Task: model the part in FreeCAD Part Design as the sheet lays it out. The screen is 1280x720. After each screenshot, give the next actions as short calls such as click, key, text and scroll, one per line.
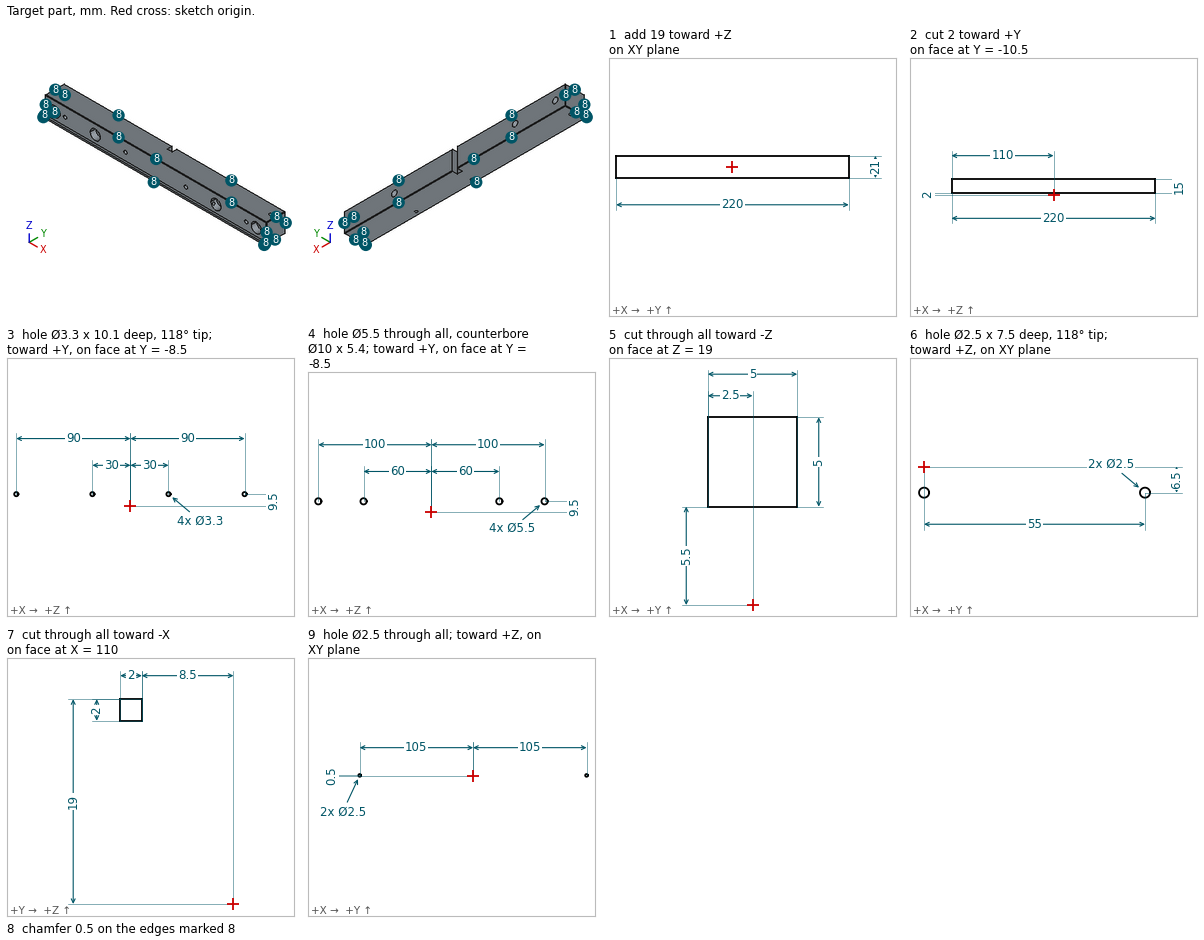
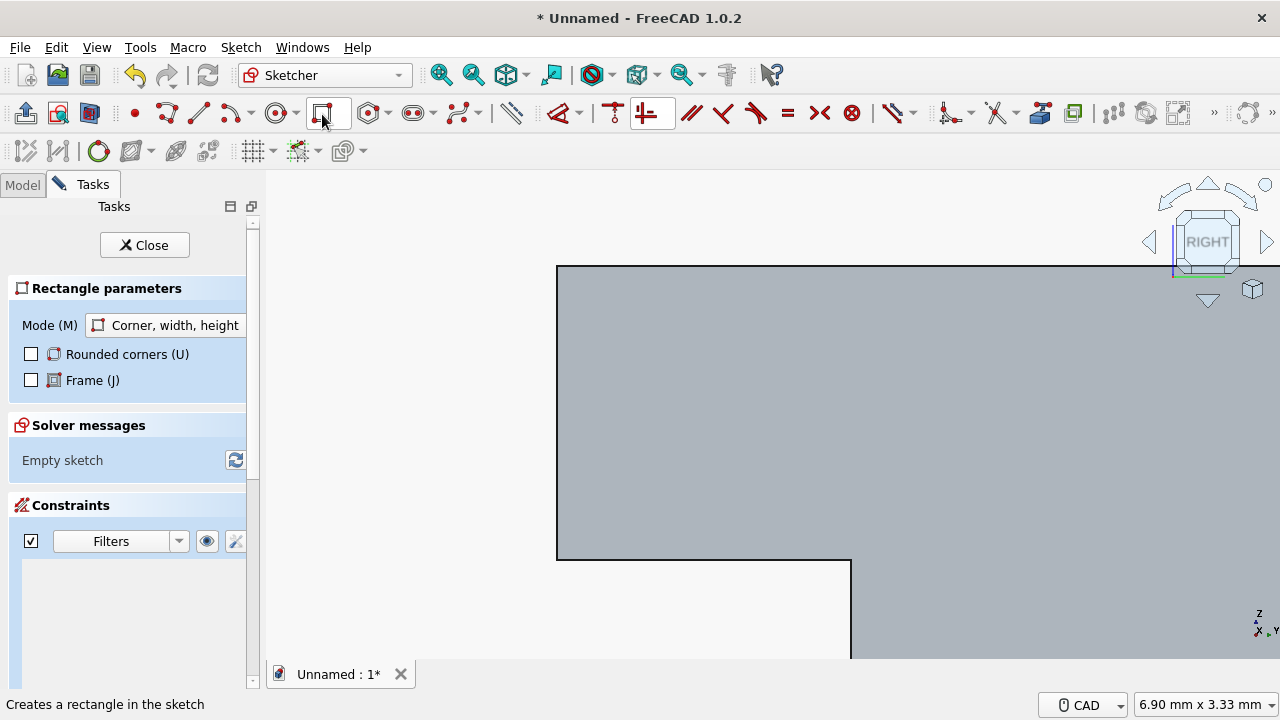
click(557, 266)
move(851, 560)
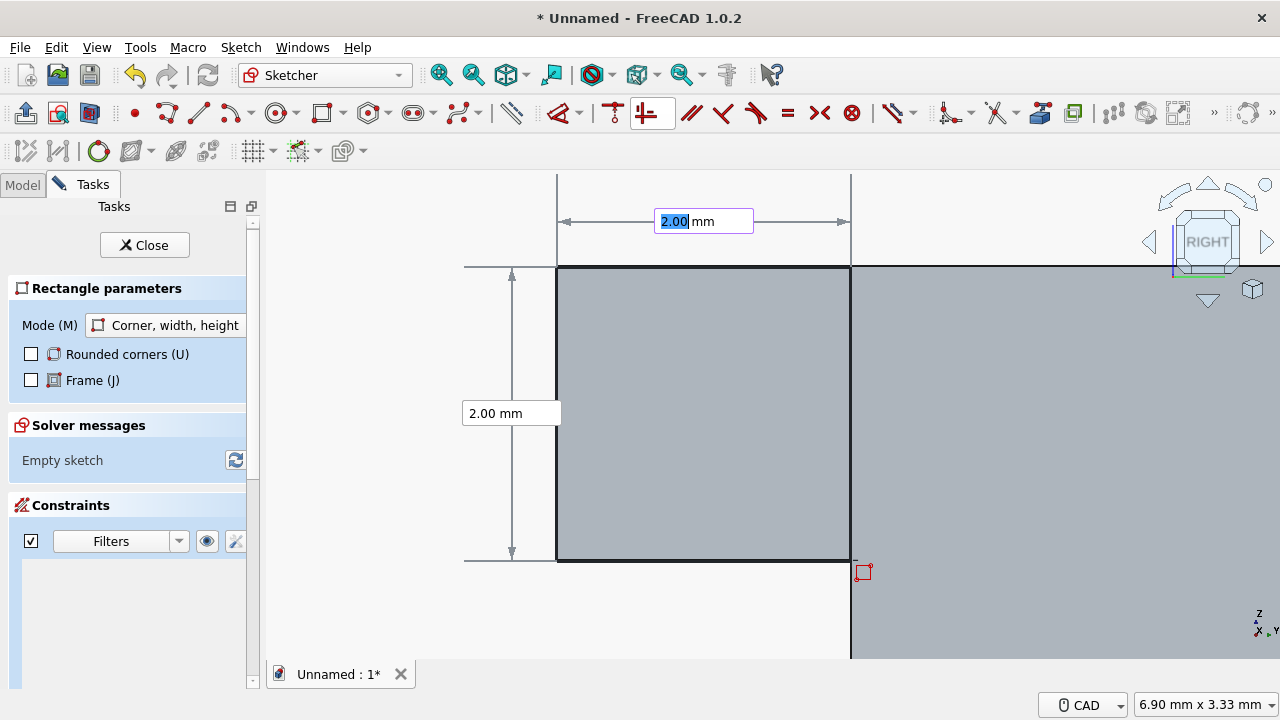
text(2)
key(Tab)
text(2)
key(Return)
key(Escape)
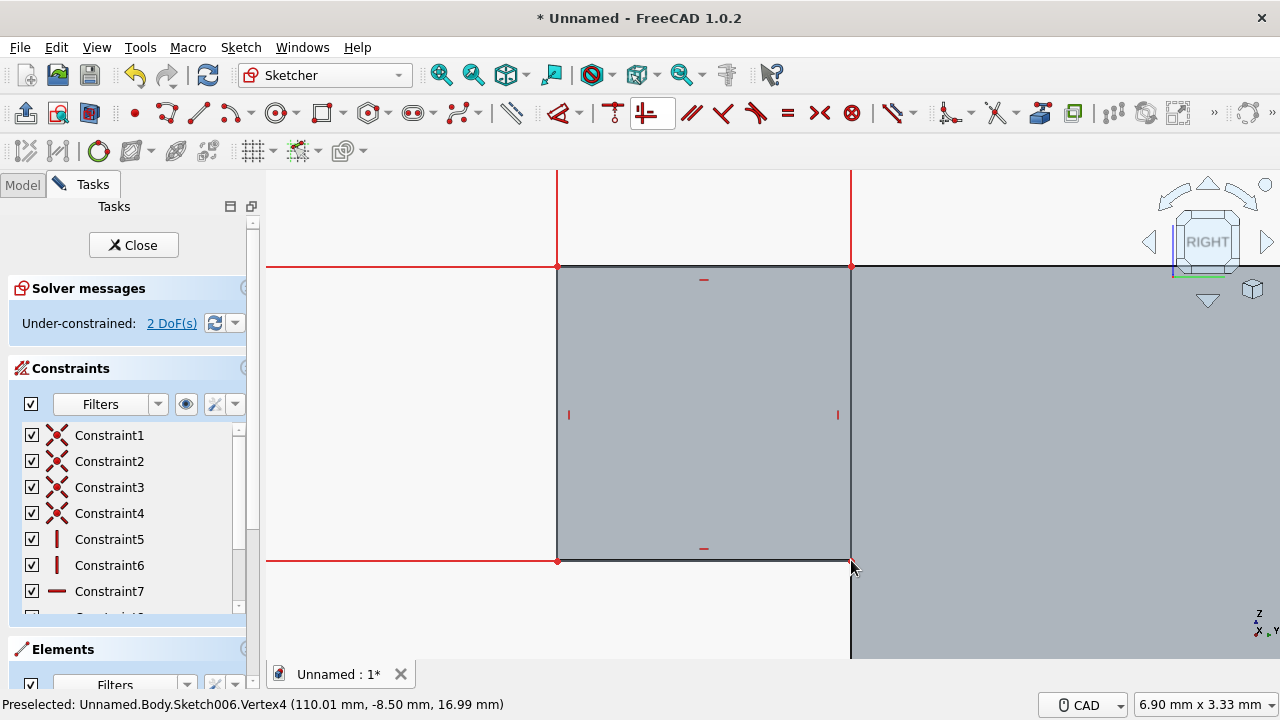
click(558, 114)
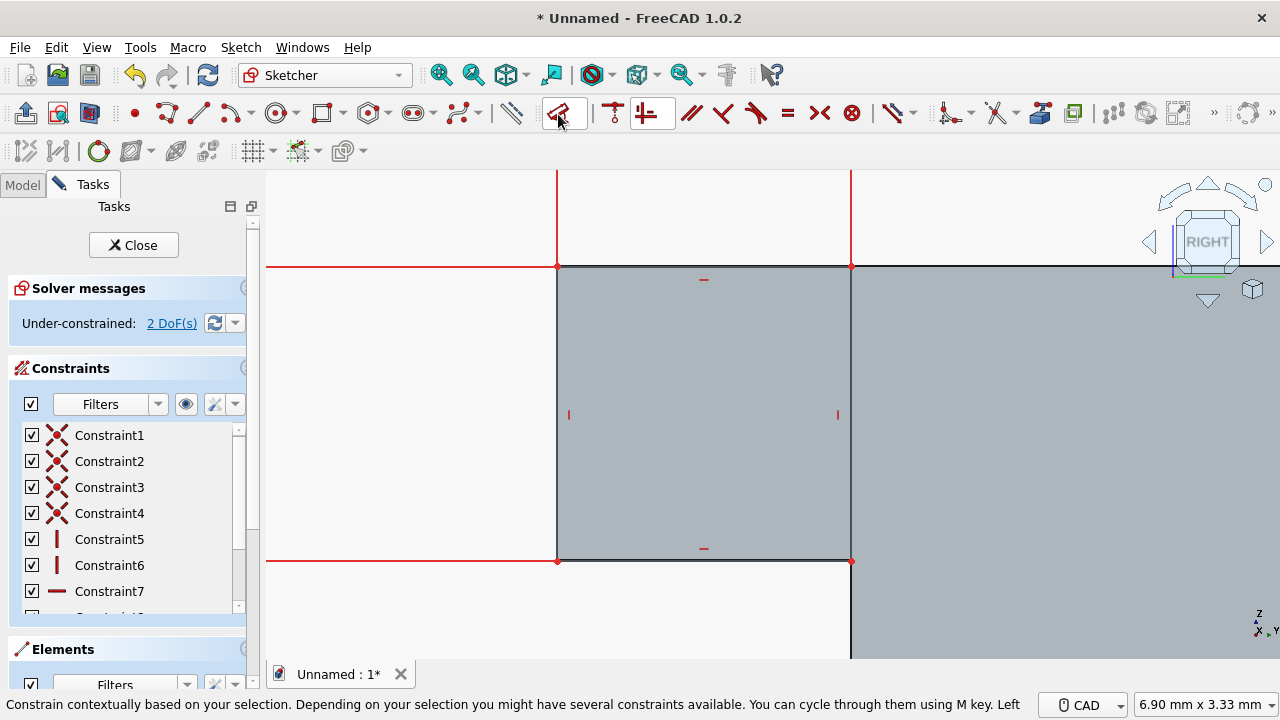
click(557, 267)
click(523, 449)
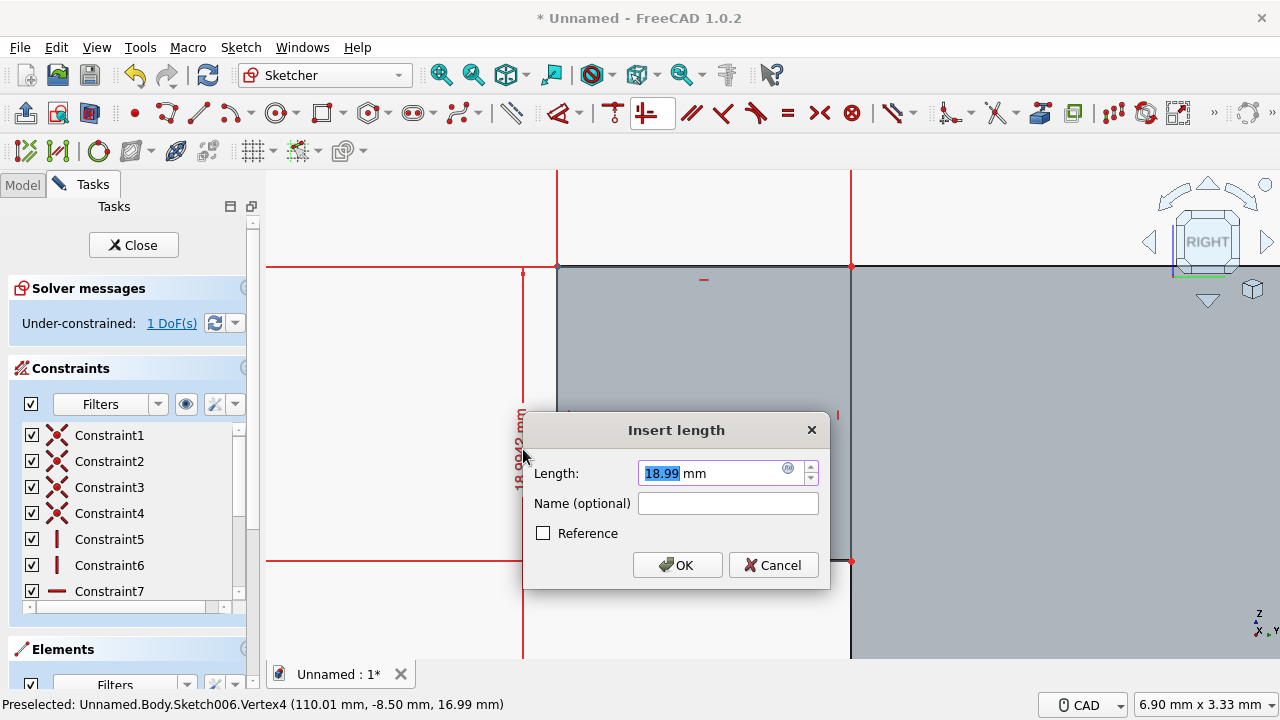
text(19)
key(Return)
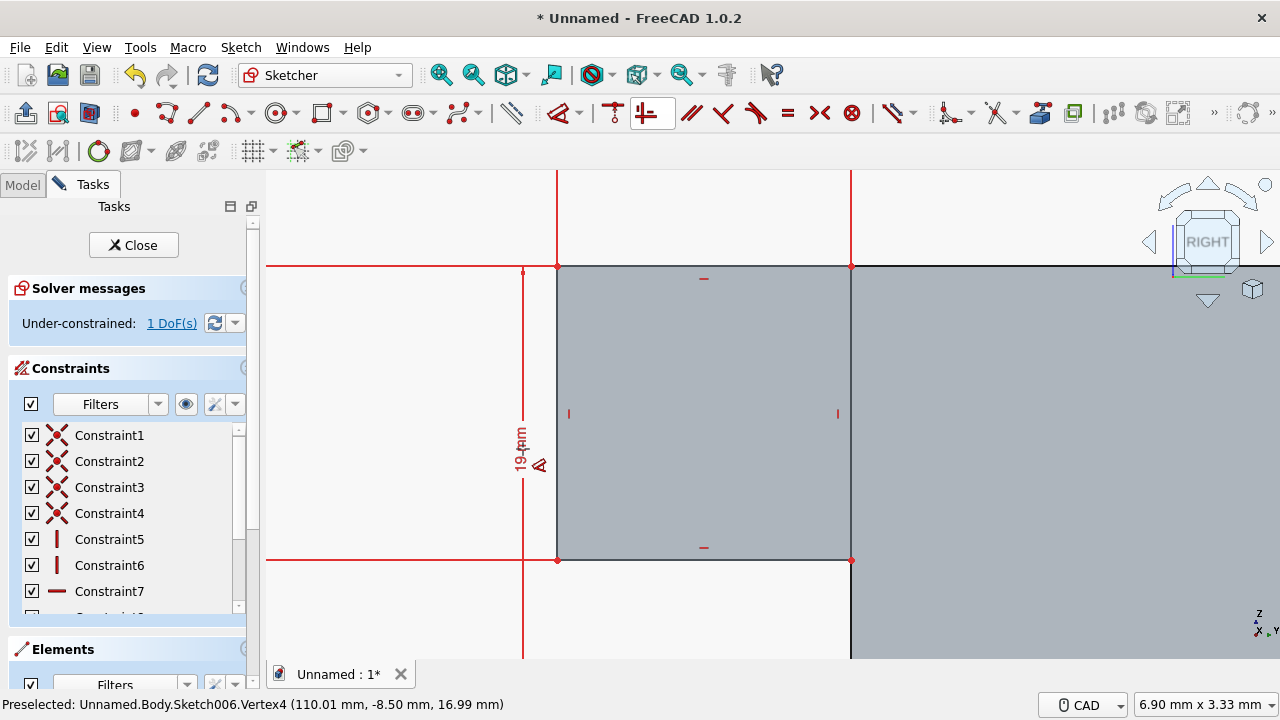
click(851, 560)
click(983, 526)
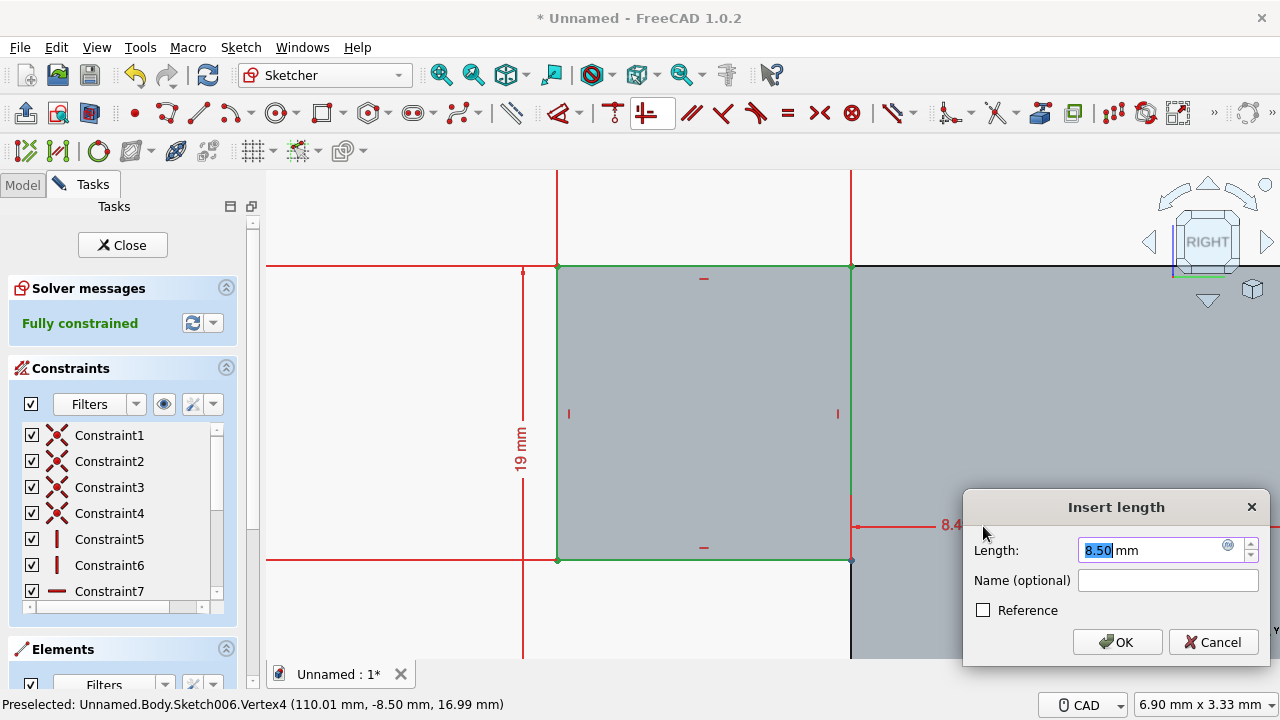
text(8.5)
key(Return)
key(Escape)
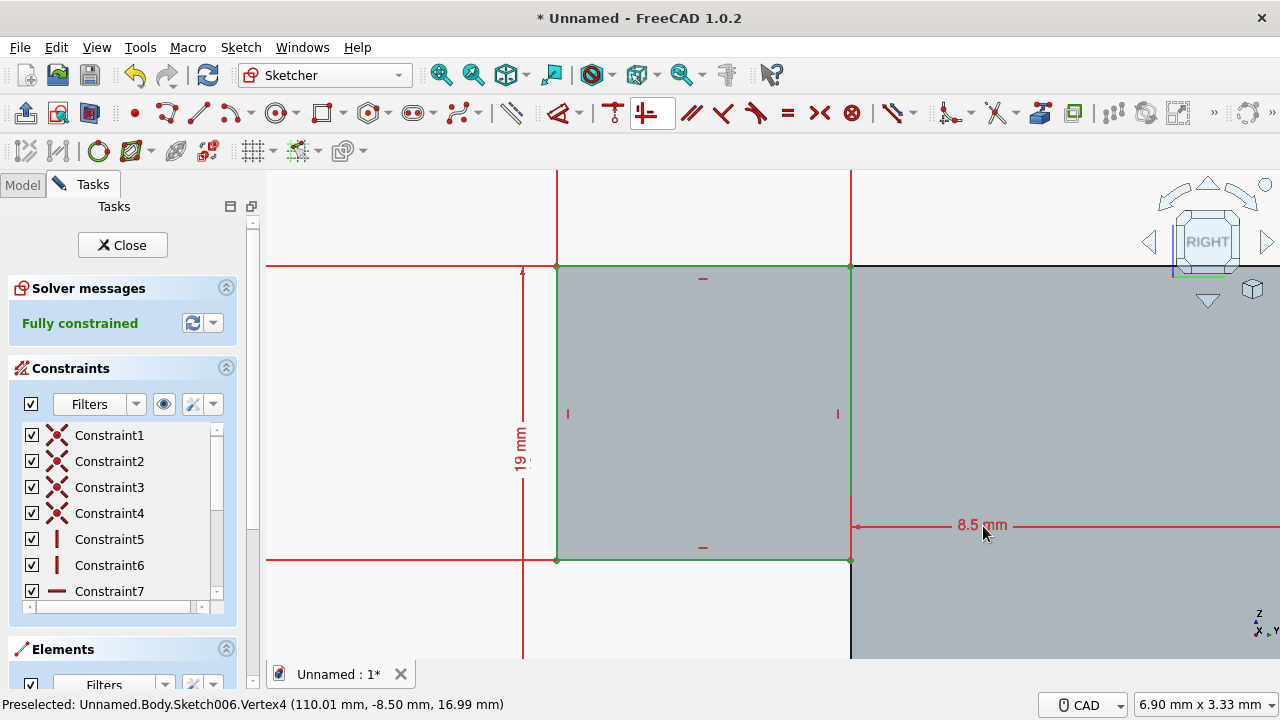
click(123, 245)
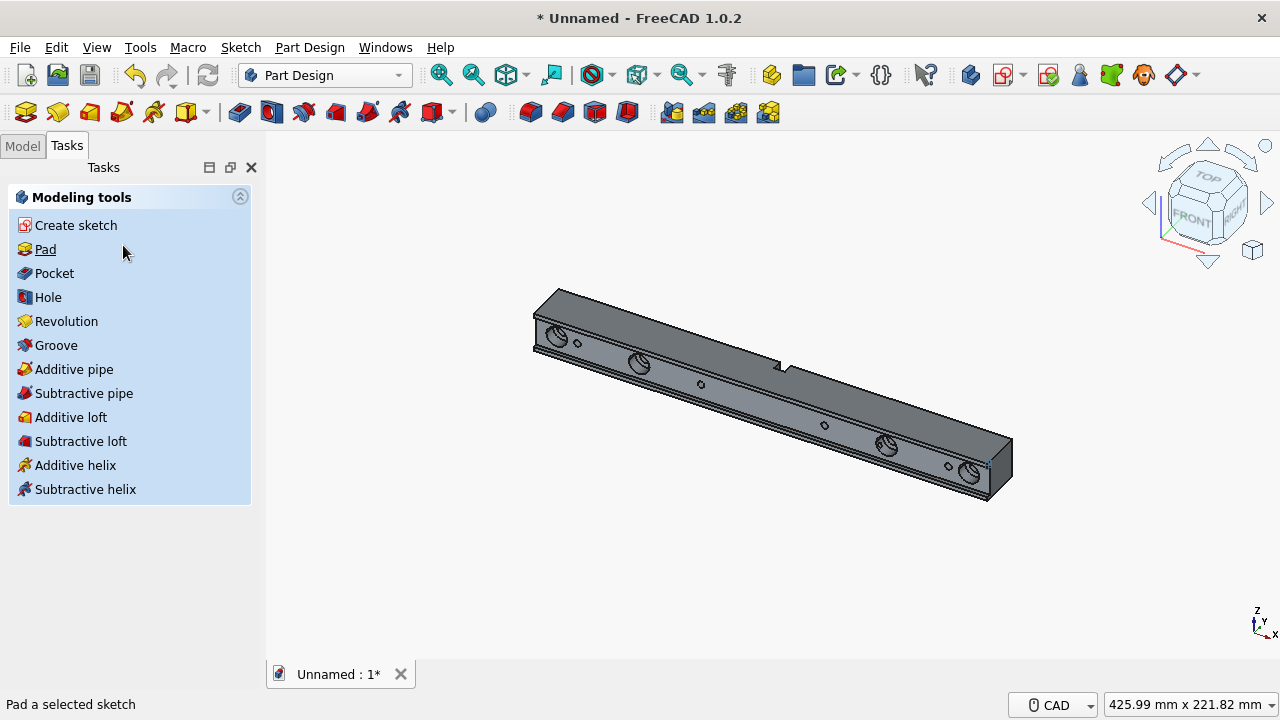
click(240, 112)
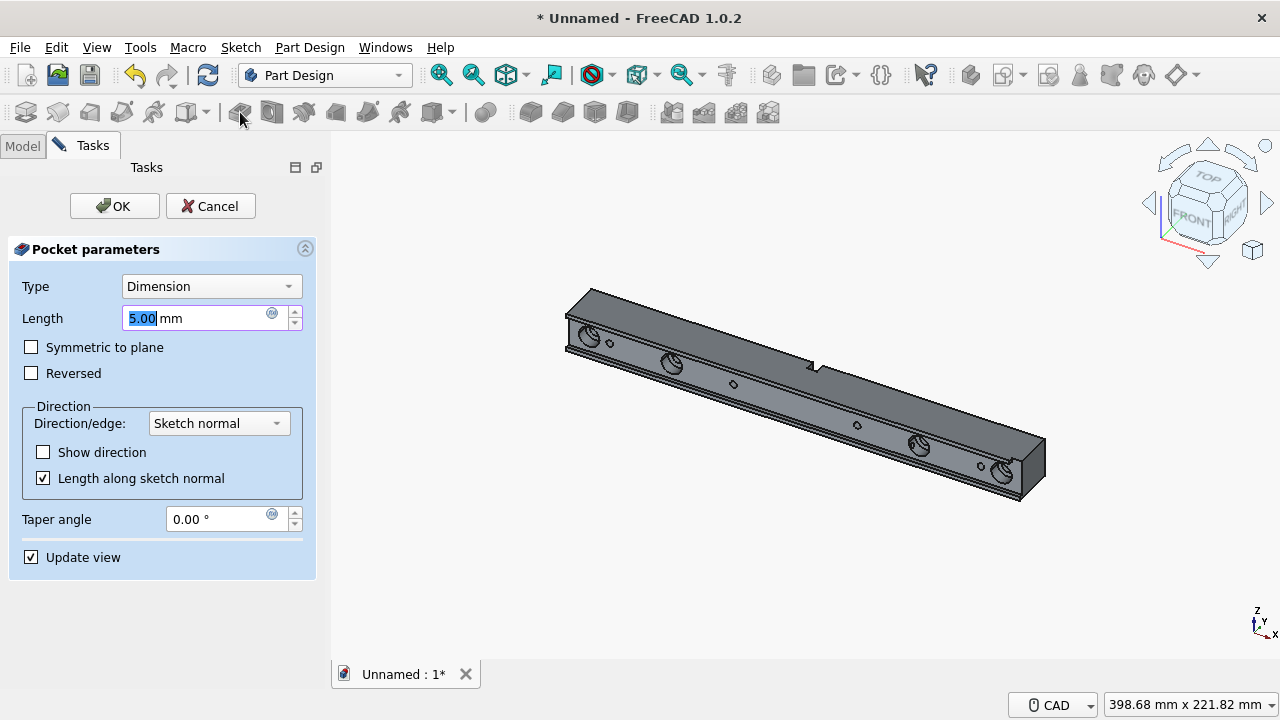
click(212, 286)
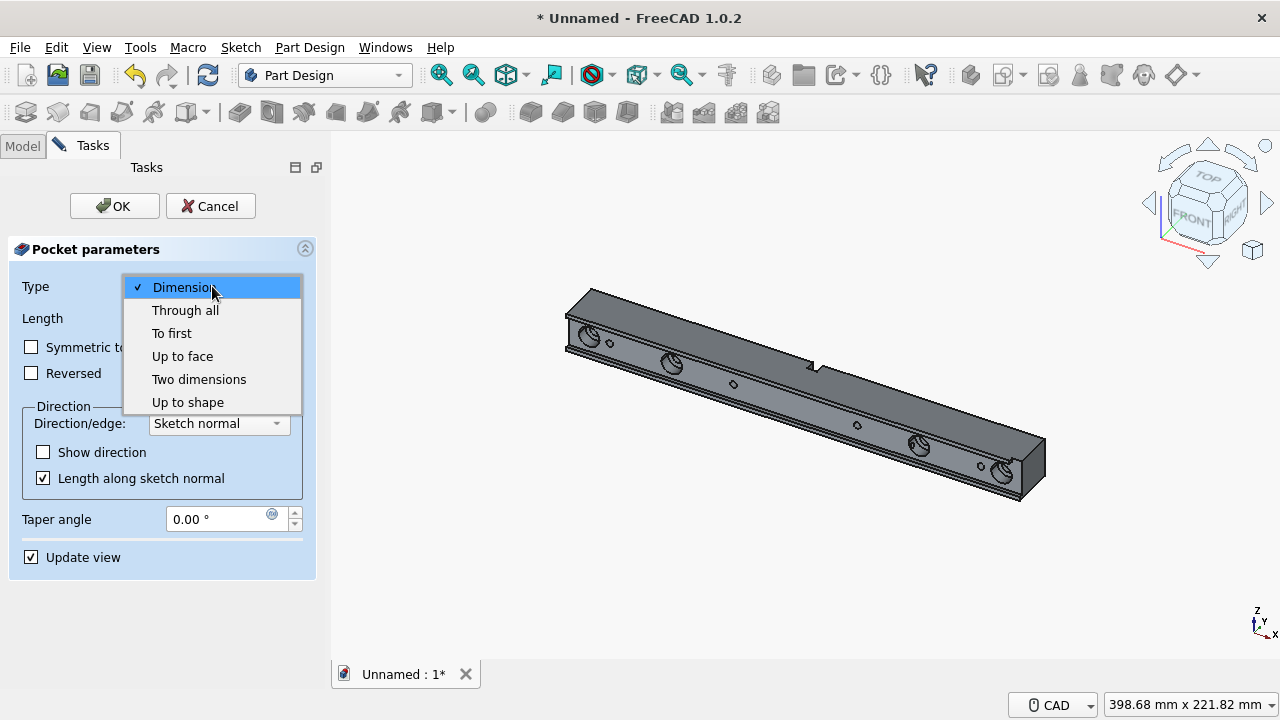
click(212, 310)